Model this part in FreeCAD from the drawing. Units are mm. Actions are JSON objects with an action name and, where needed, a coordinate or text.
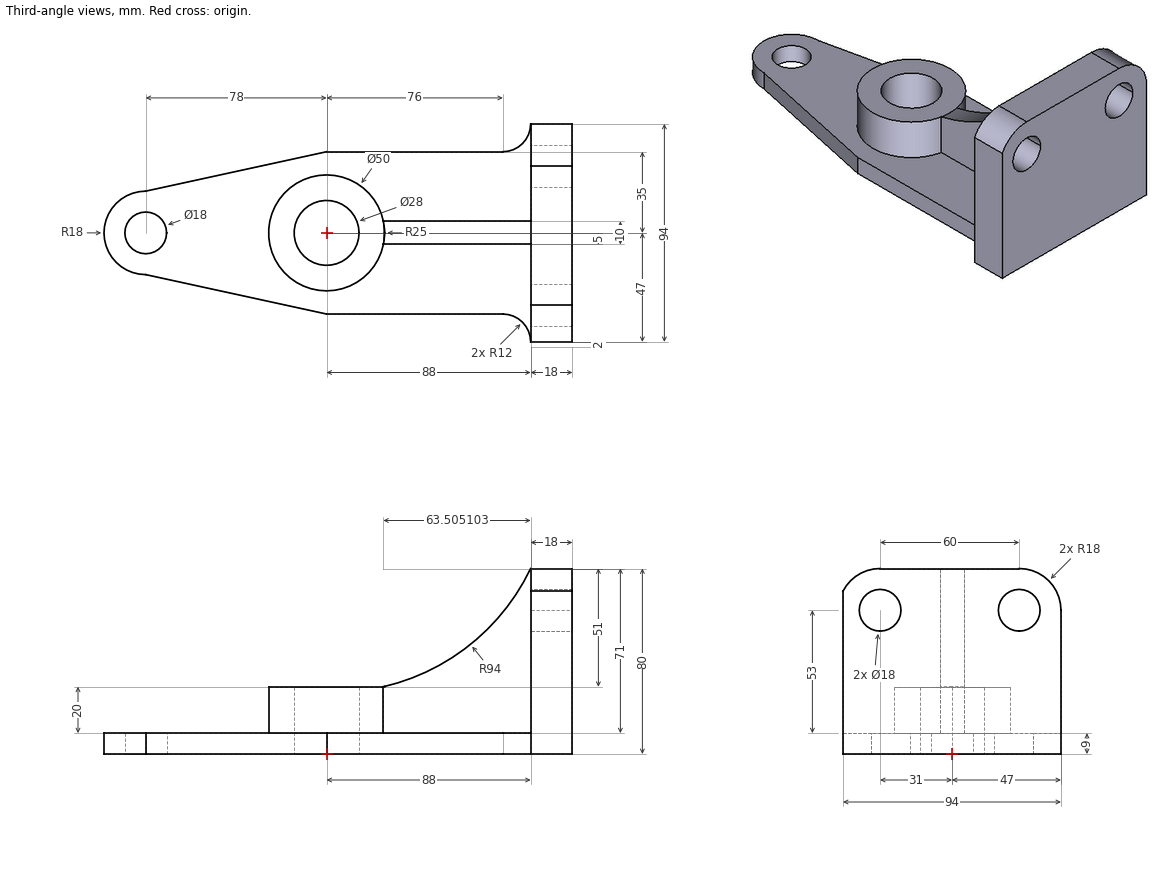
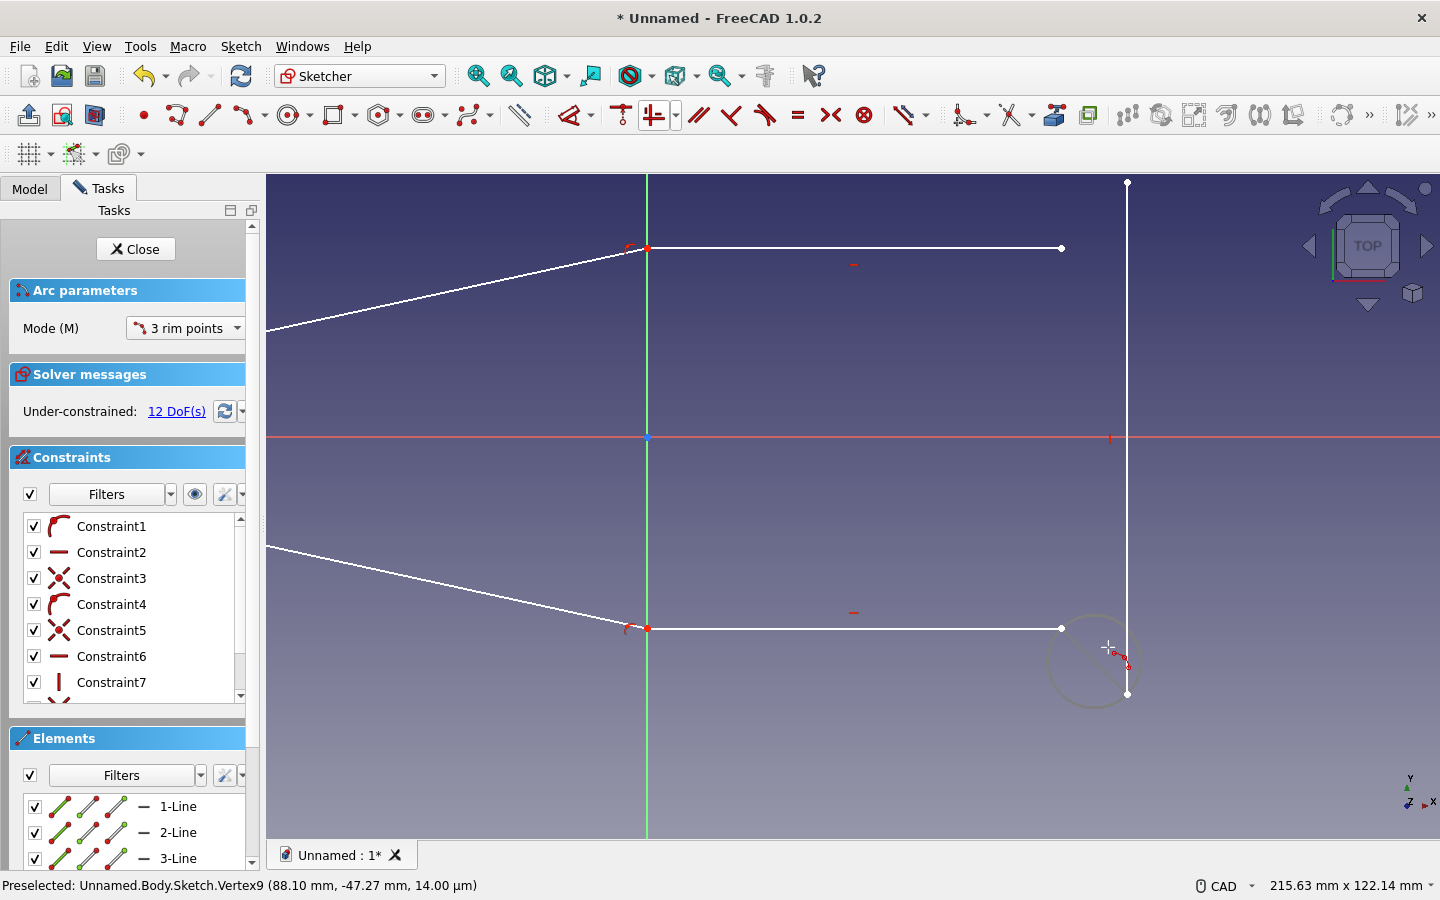
{"action": "left_click", "coordinate": [1107, 647]}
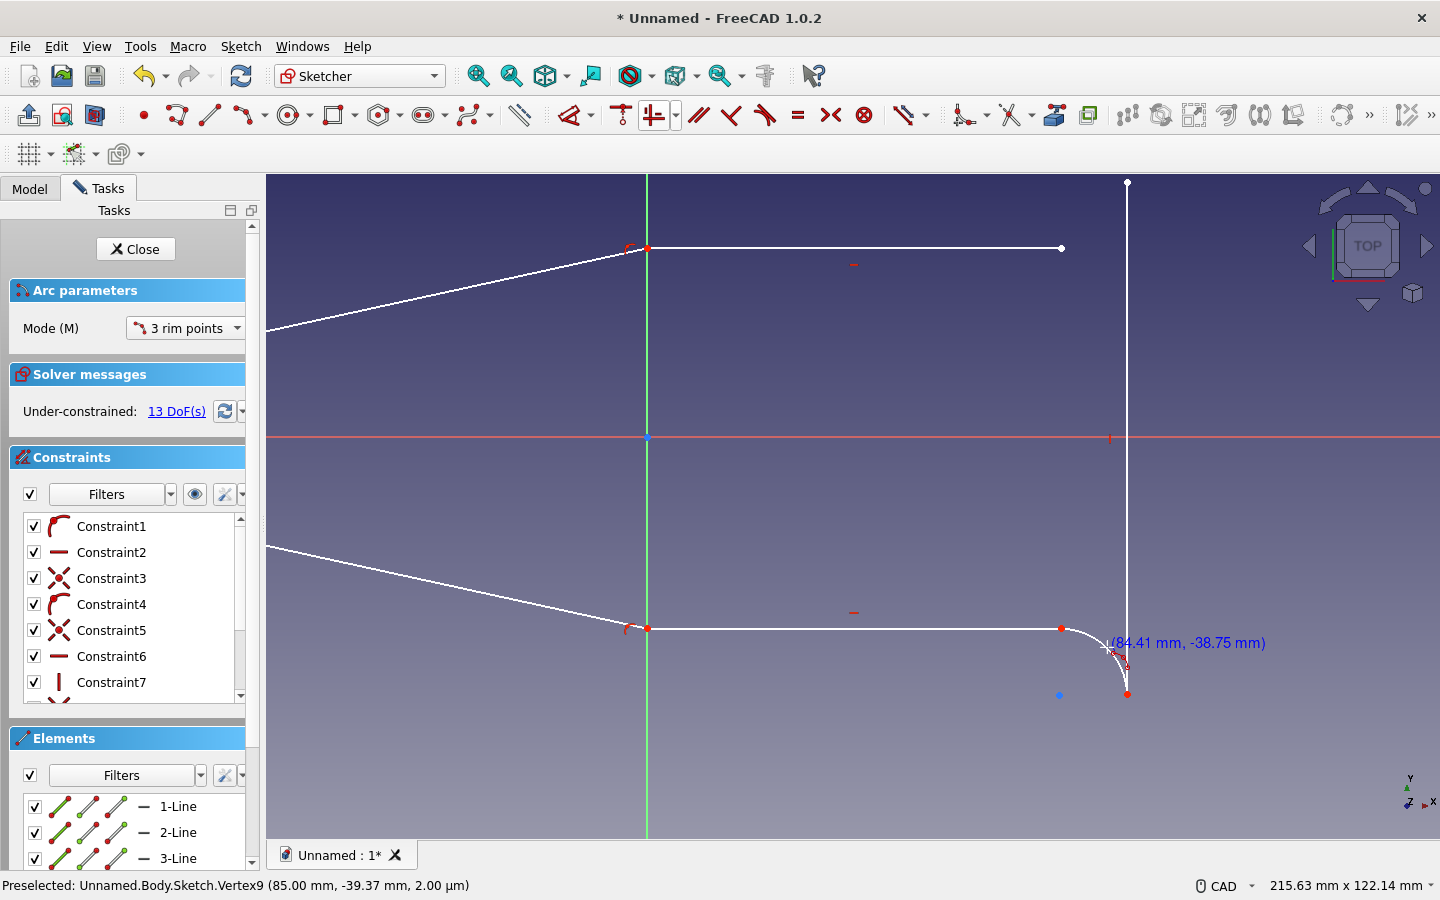
{"action": "scroll", "coordinate": [1108, 648], "scroll_direction": "down", "scroll_amount": 2}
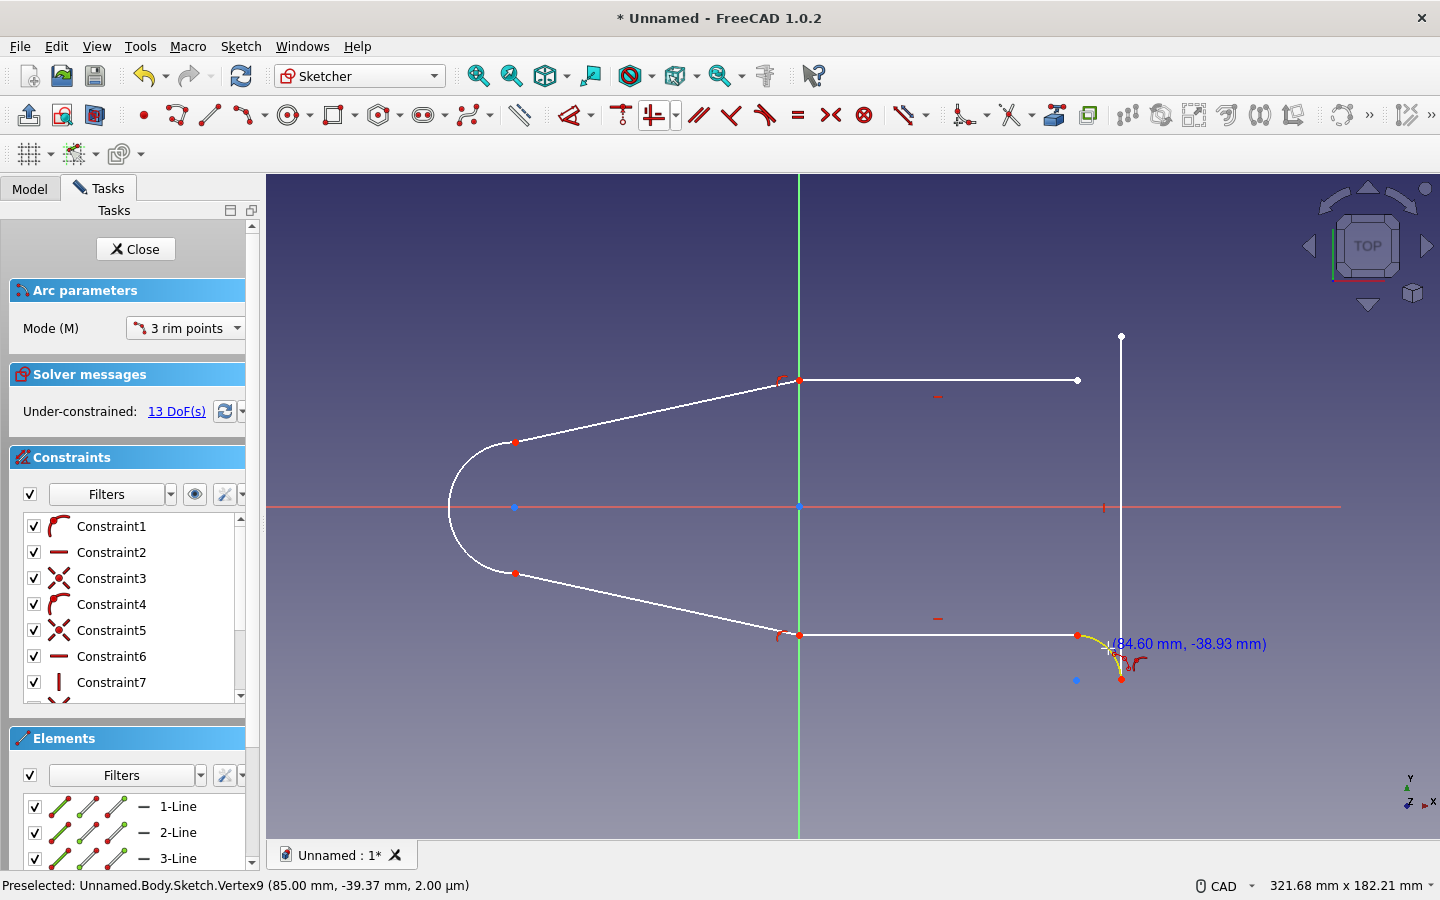
{"action": "left_click", "coordinate": [1121, 336]}
{"action": "left_click", "coordinate": [1077, 380]}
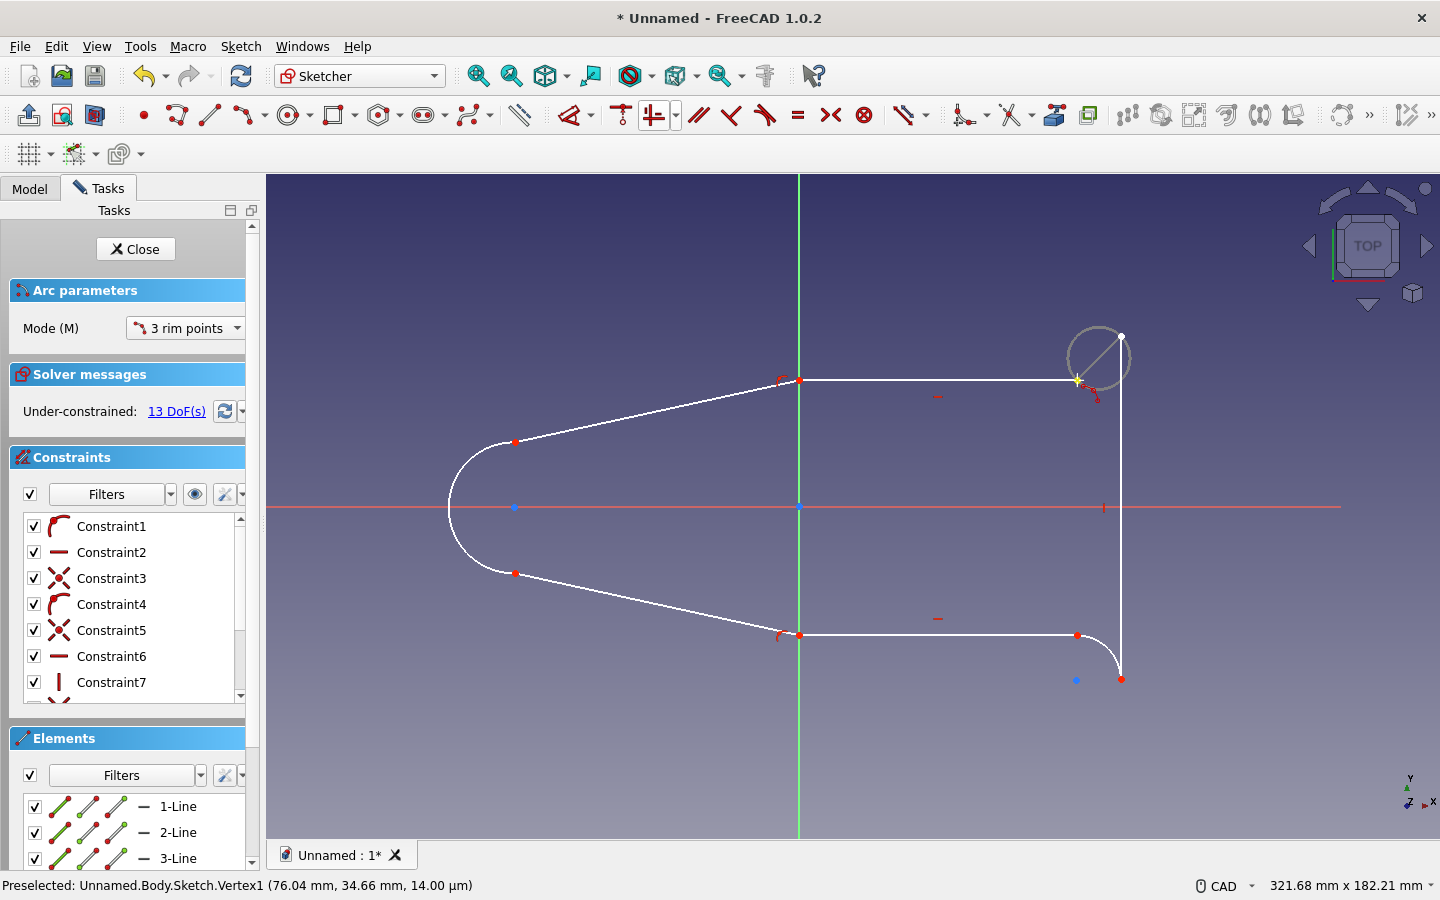
{"action": "scroll", "coordinate": [1108, 366], "scroll_direction": "up", "scroll_amount": 2}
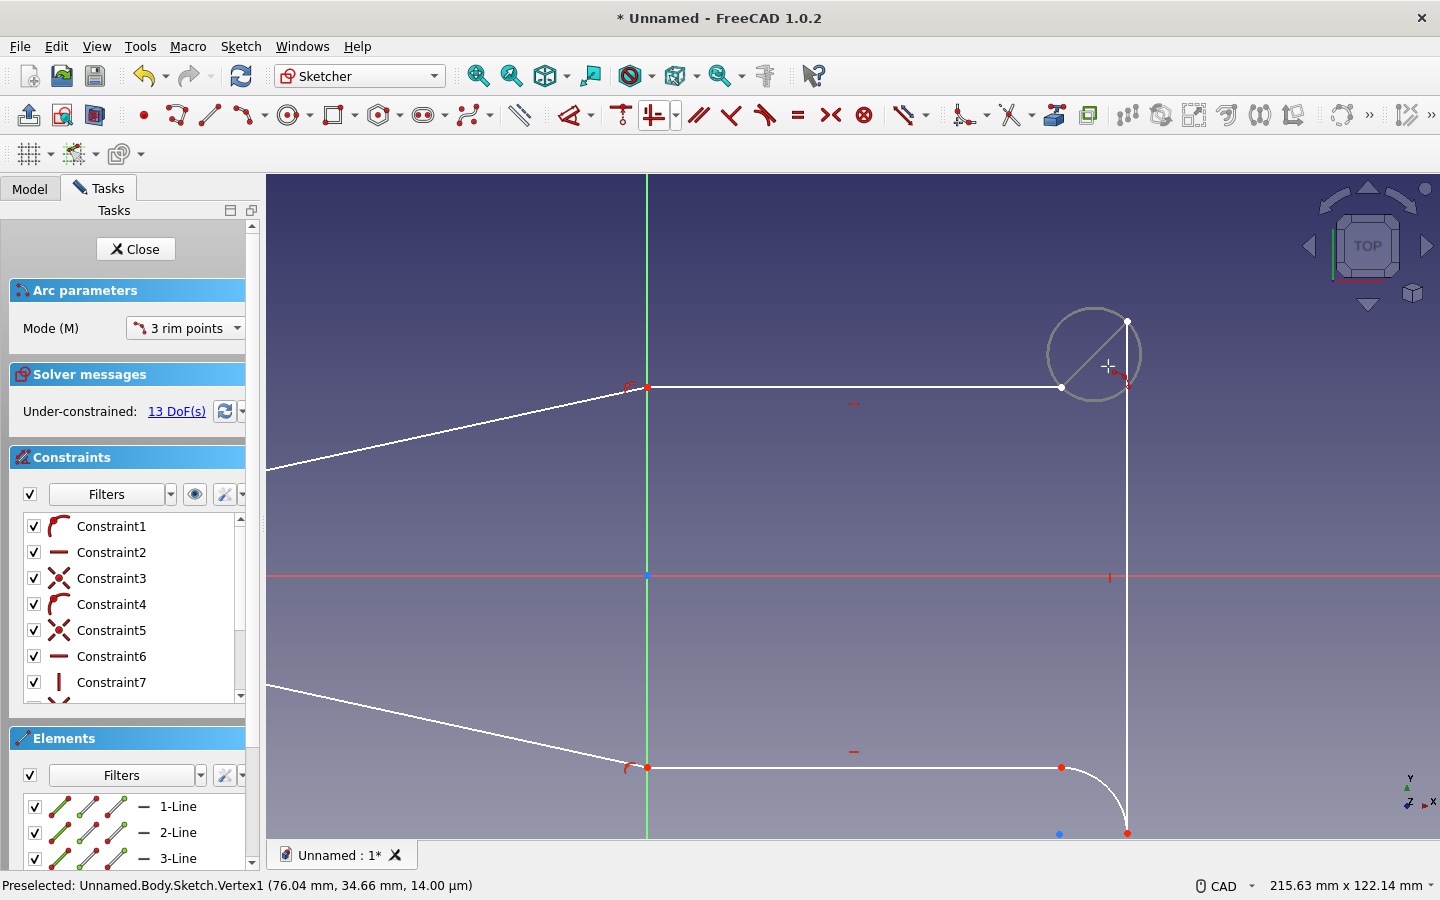
{"action": "left_click", "coordinate": [1107, 366]}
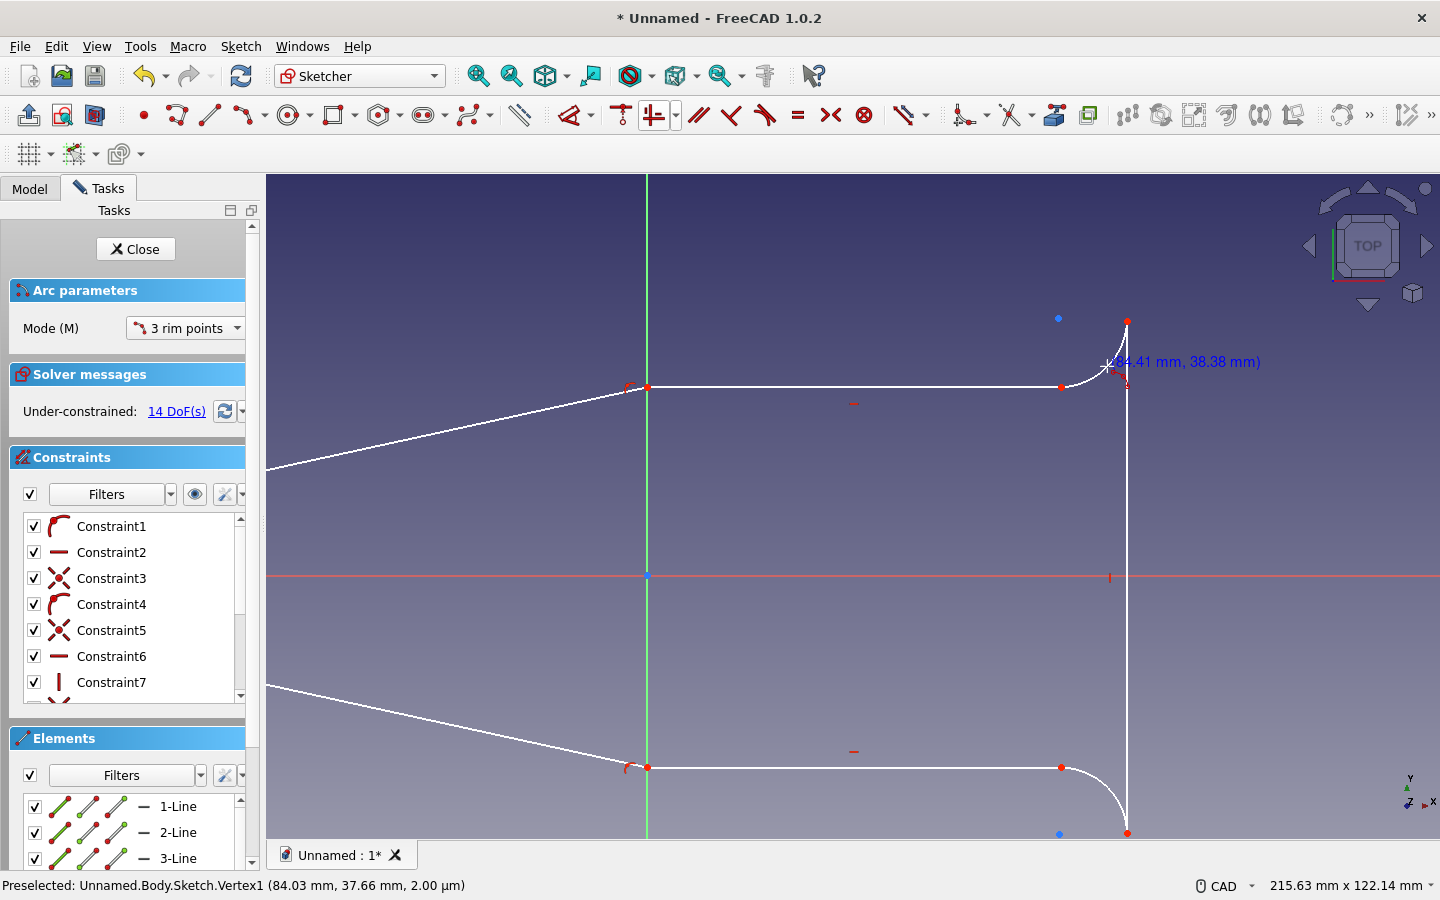
{"action": "left_click", "coordinate": [288, 116]}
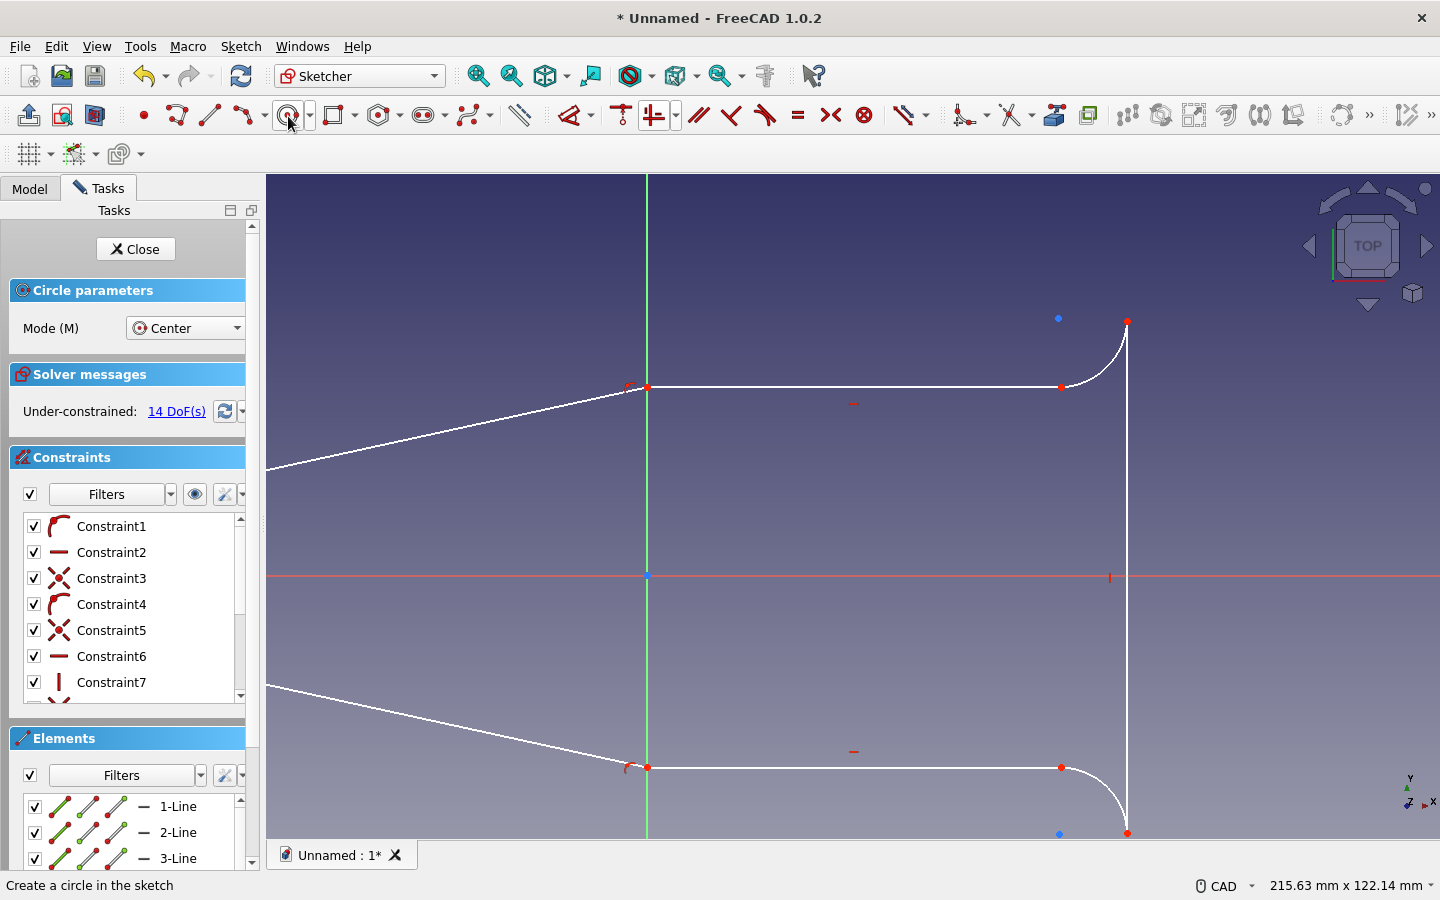
{"action": "scroll", "coordinate": [1108, 365], "scroll_direction": "down", "scroll_amount": 2}